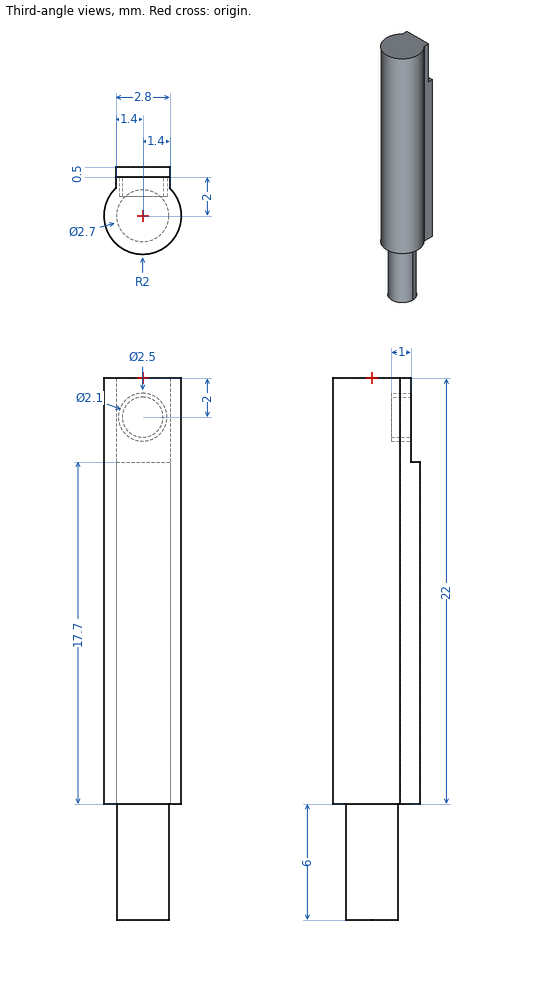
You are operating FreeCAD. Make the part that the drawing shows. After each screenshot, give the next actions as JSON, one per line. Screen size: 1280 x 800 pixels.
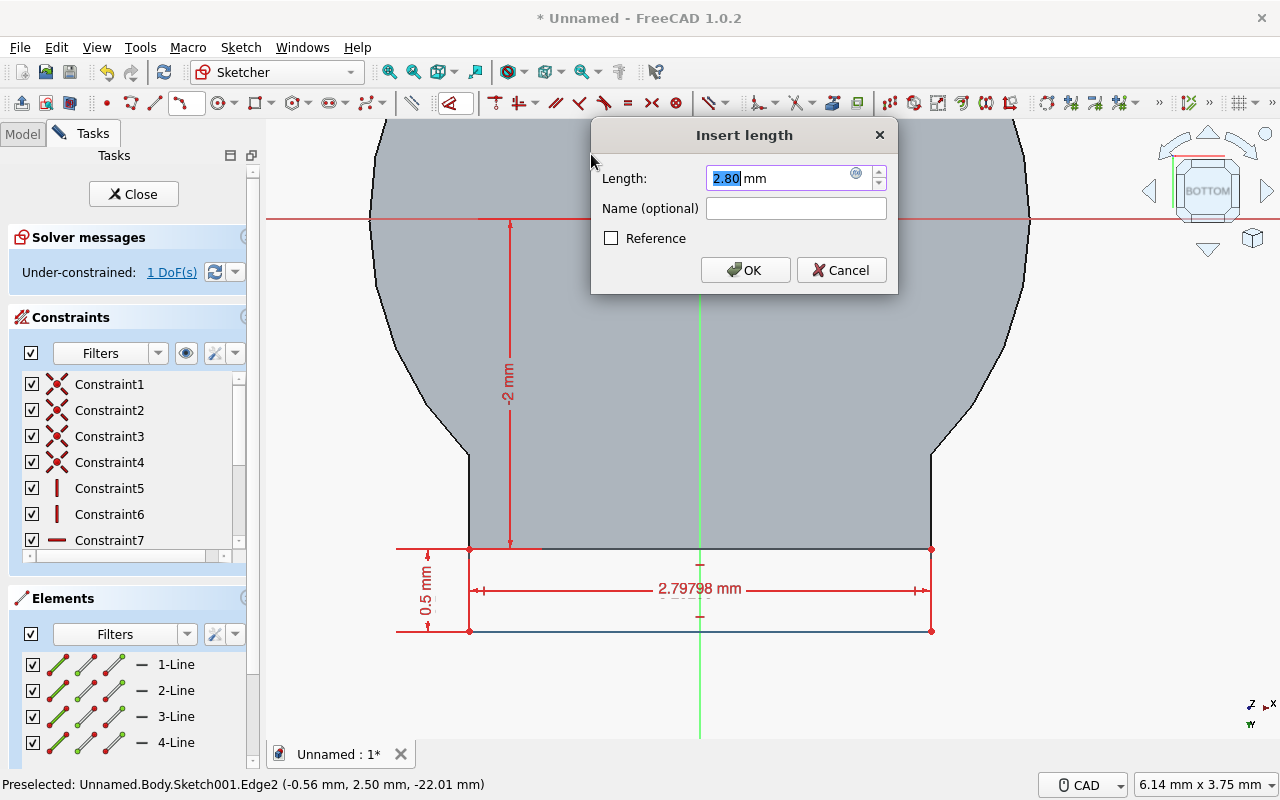
{"action": "type", "text": "2.8"}
{"action": "key", "text": "Return"}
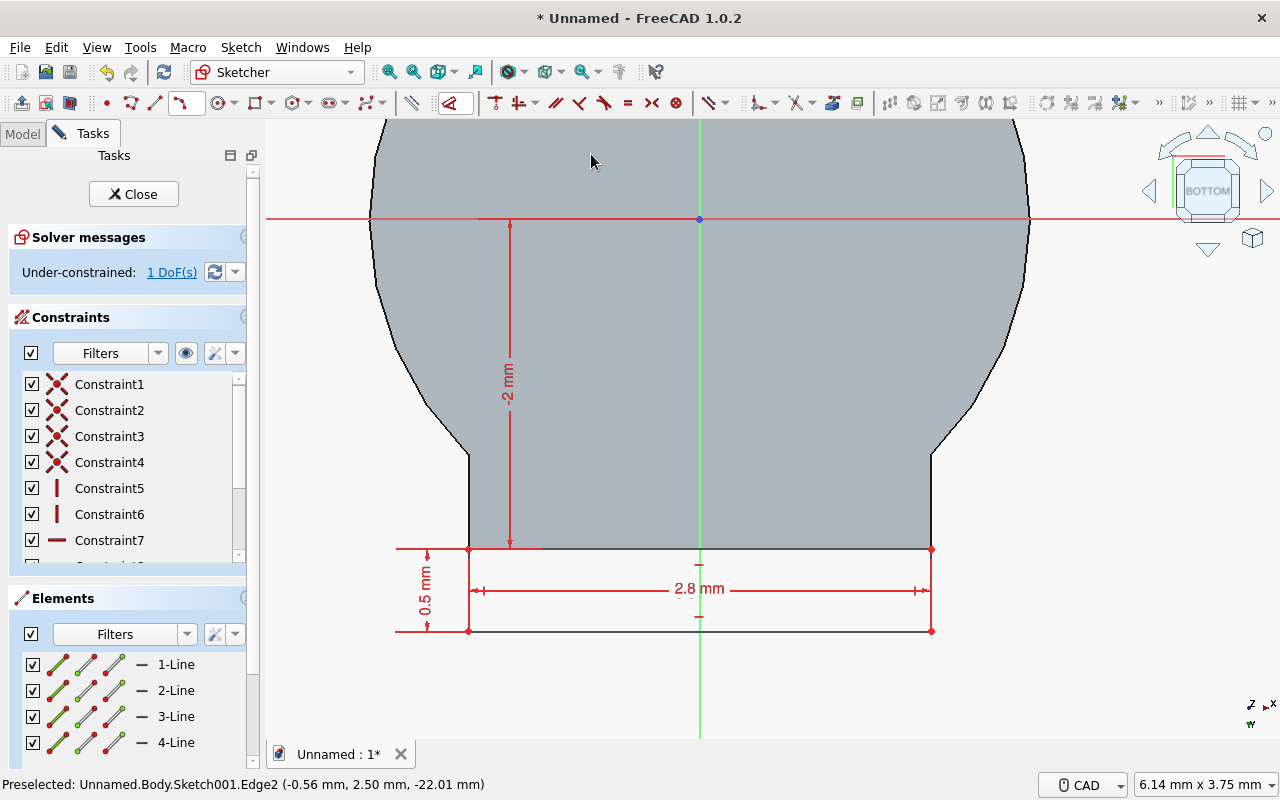
{"action": "left_click", "coordinate": [469, 549]}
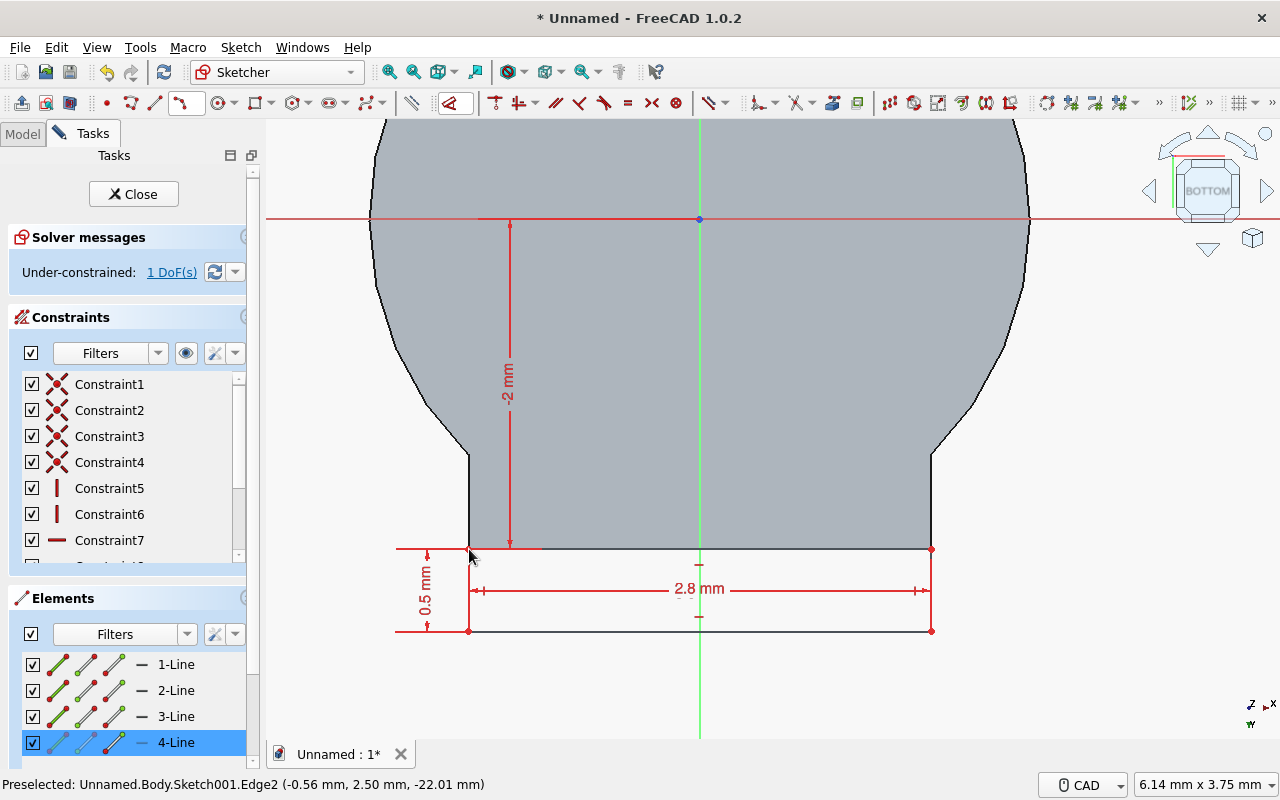
{"action": "left_click", "coordinate": [468, 104]}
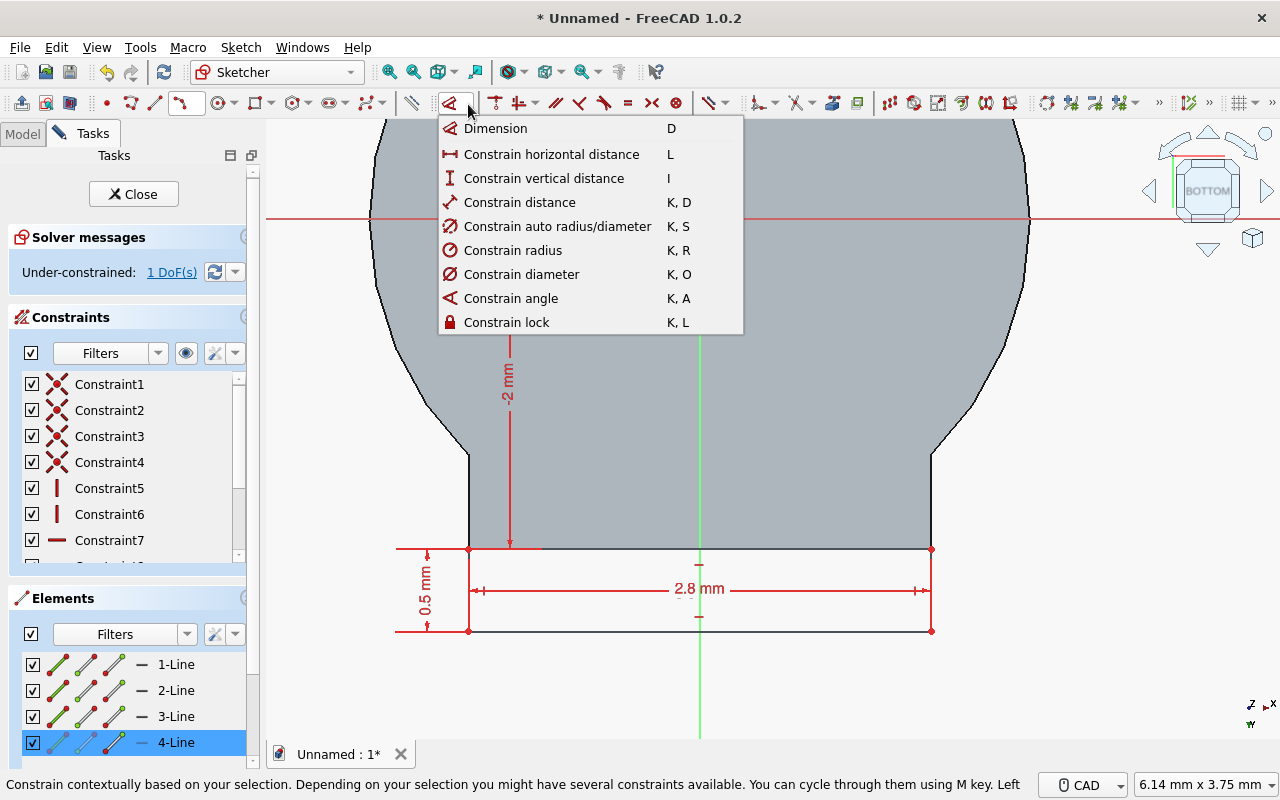
{"action": "left_click", "coordinate": [591, 154]}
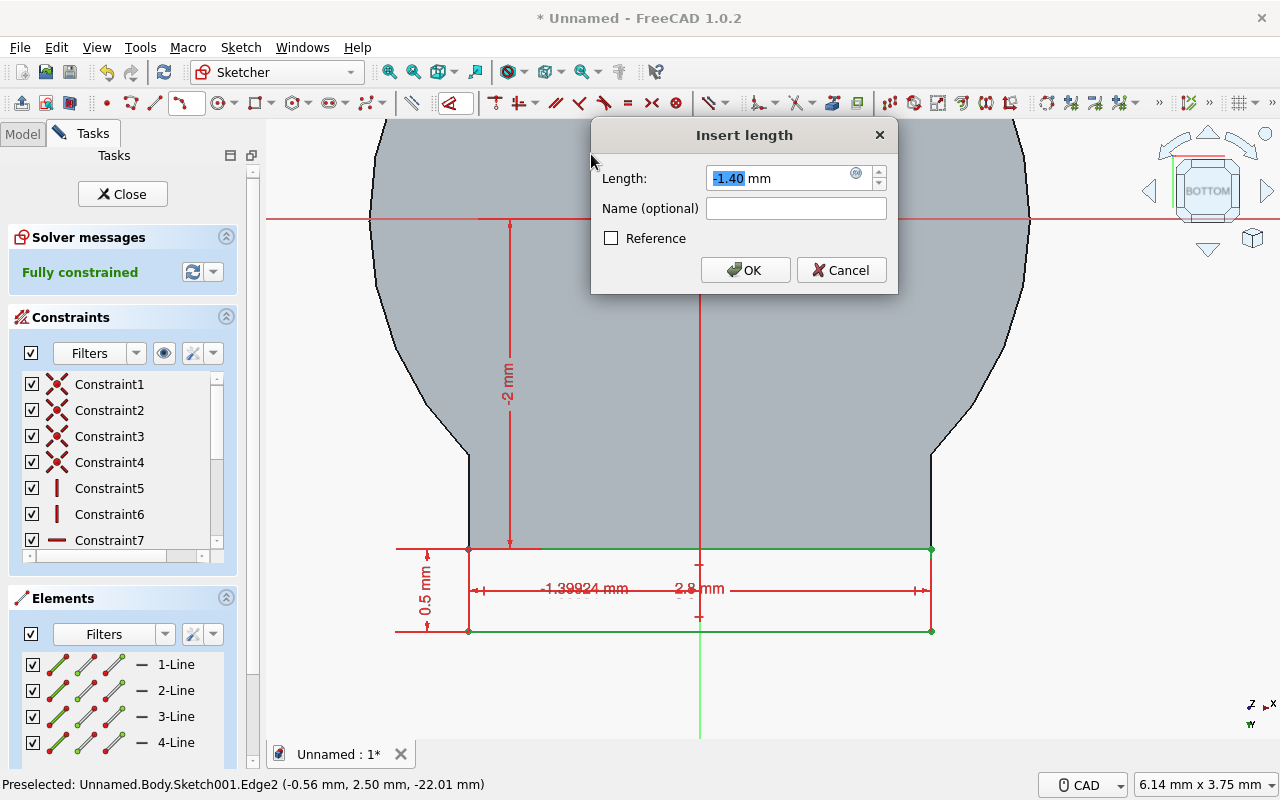
{"action": "type", "text": "-1.4"}
{"action": "key", "text": "Return"}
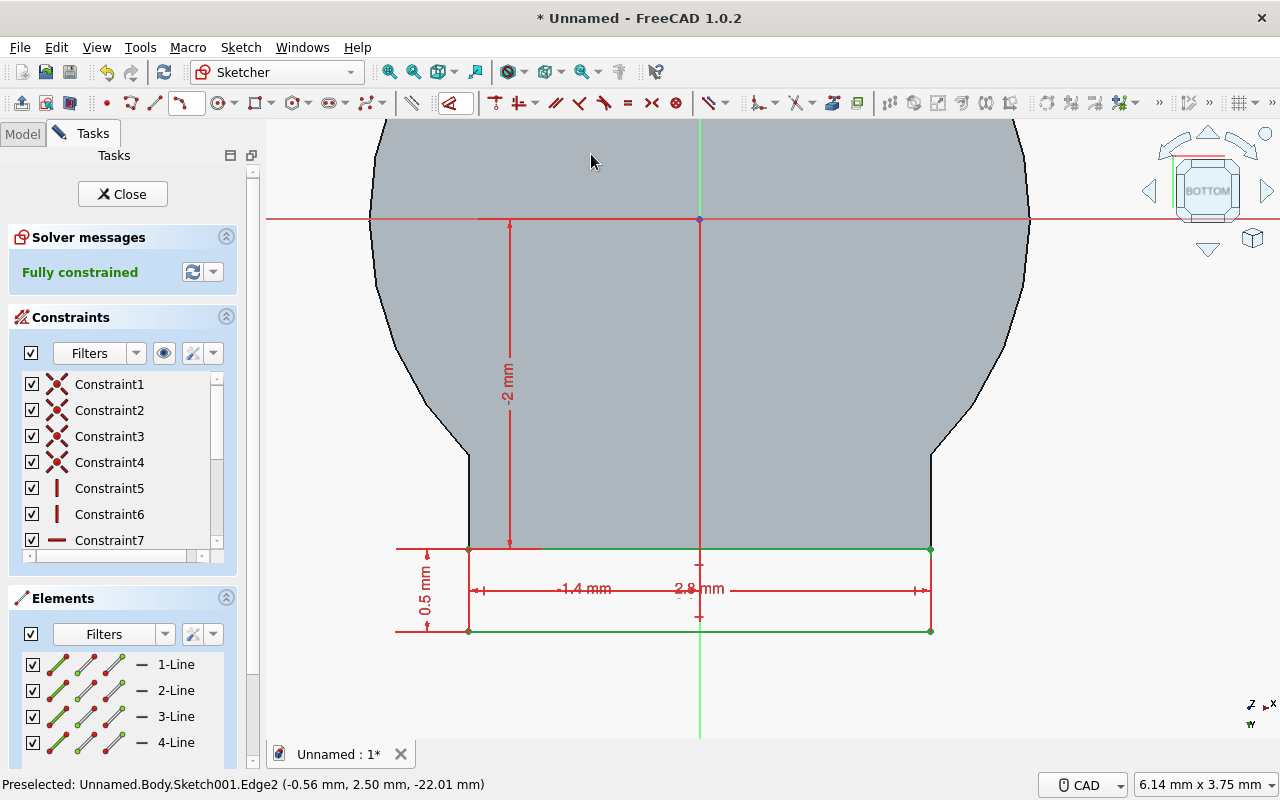
{"action": "left_click", "coordinate": [123, 194]}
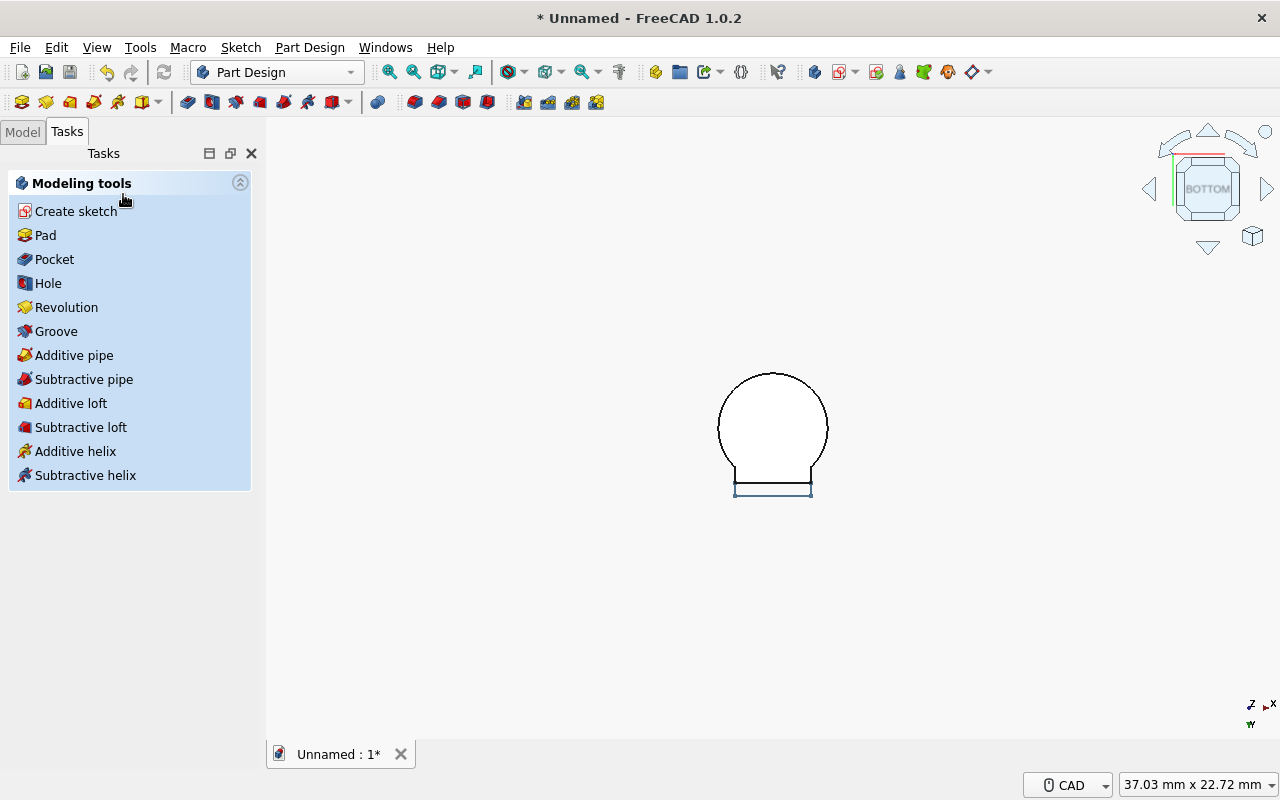
{"action": "left_click", "coordinate": [22, 102]}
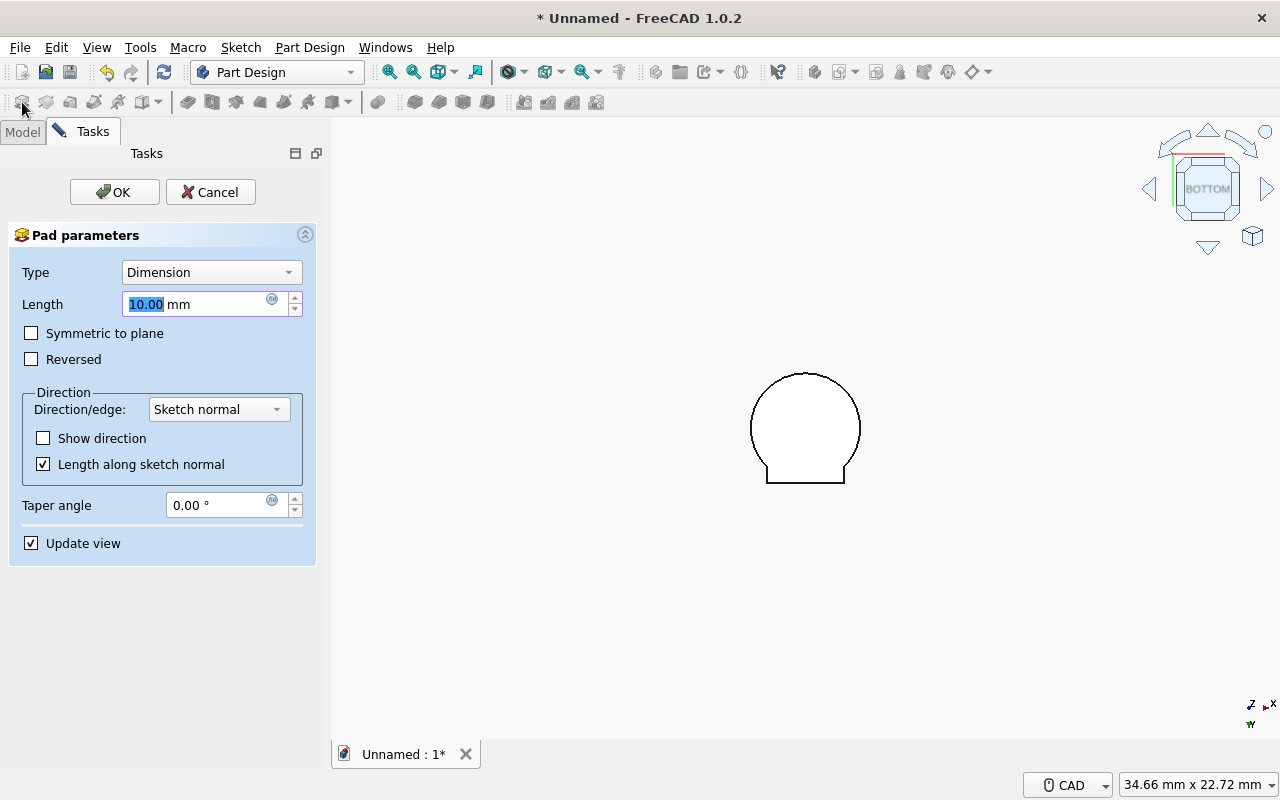
{"action": "type", "text": "17.7"}
{"action": "key", "text": "Tab"}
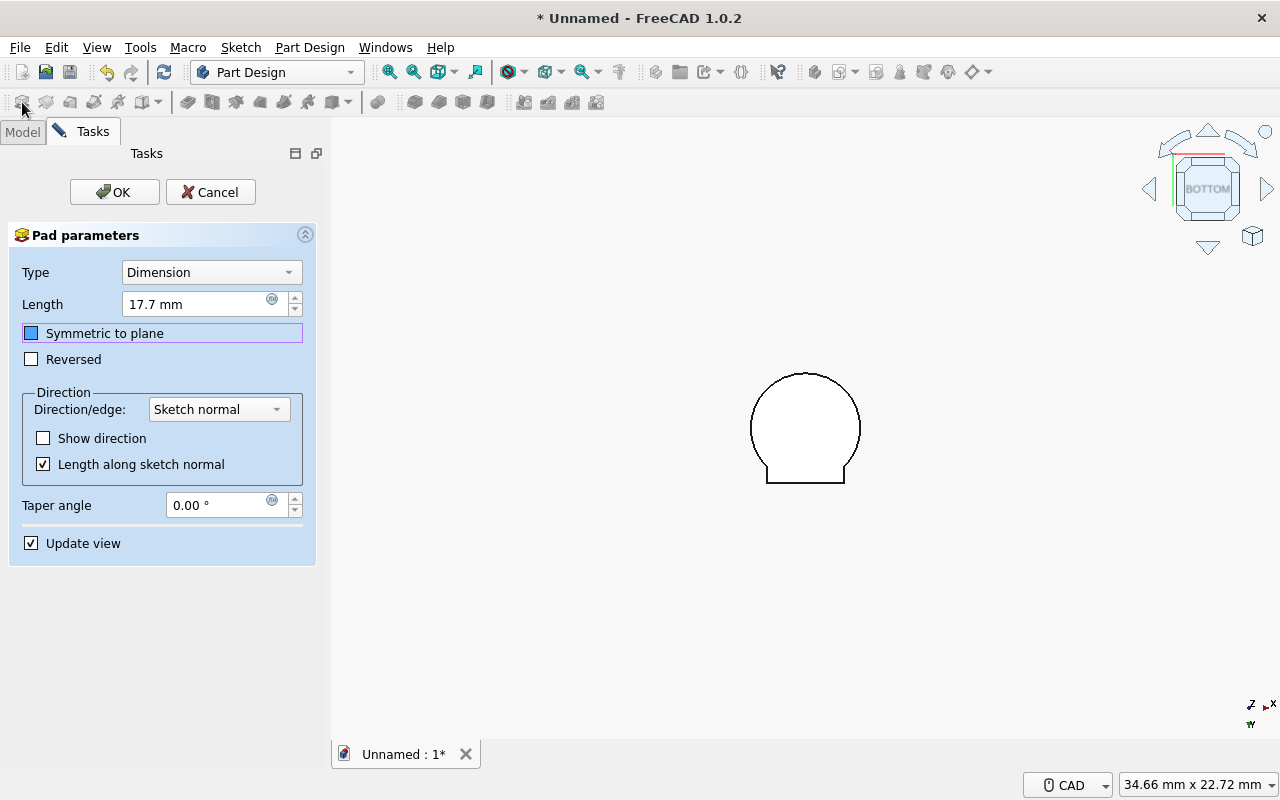
{"action": "left_click", "coordinate": [30, 359]}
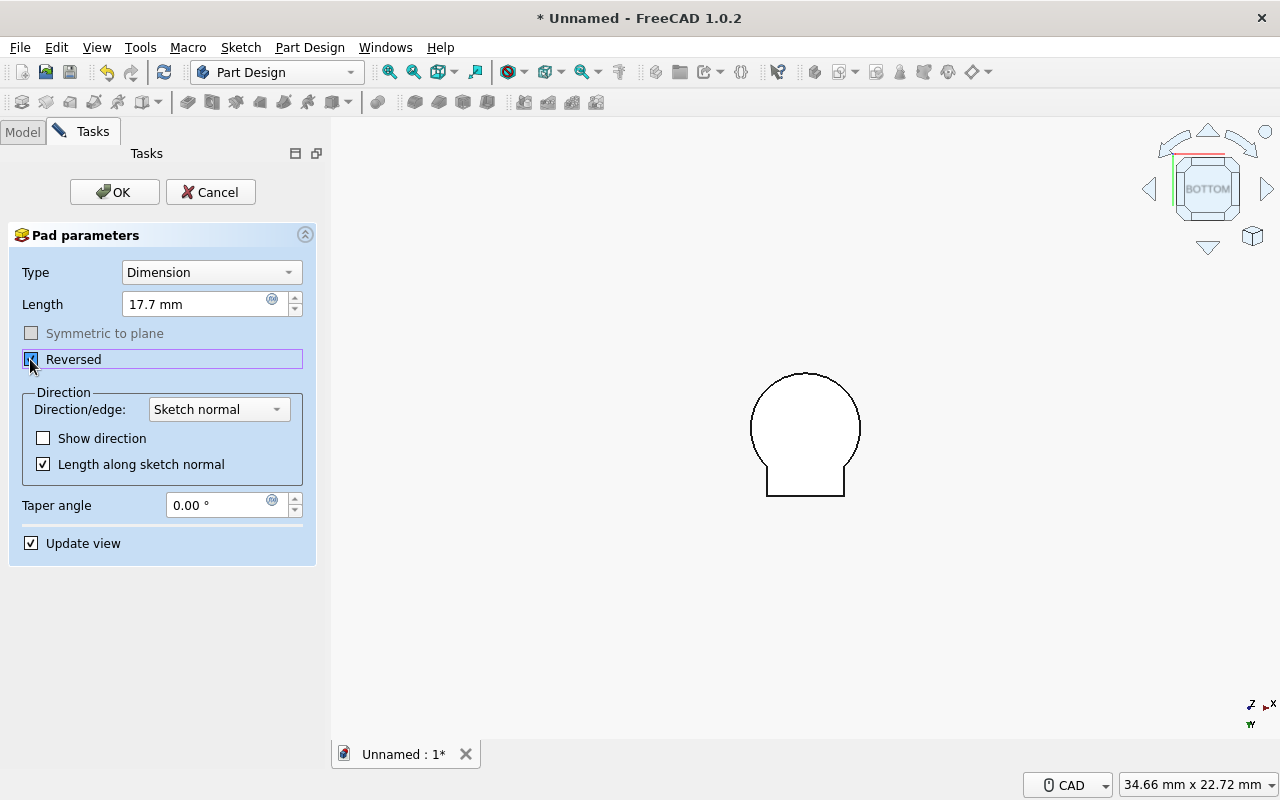
{"action": "left_click", "coordinate": [115, 192]}